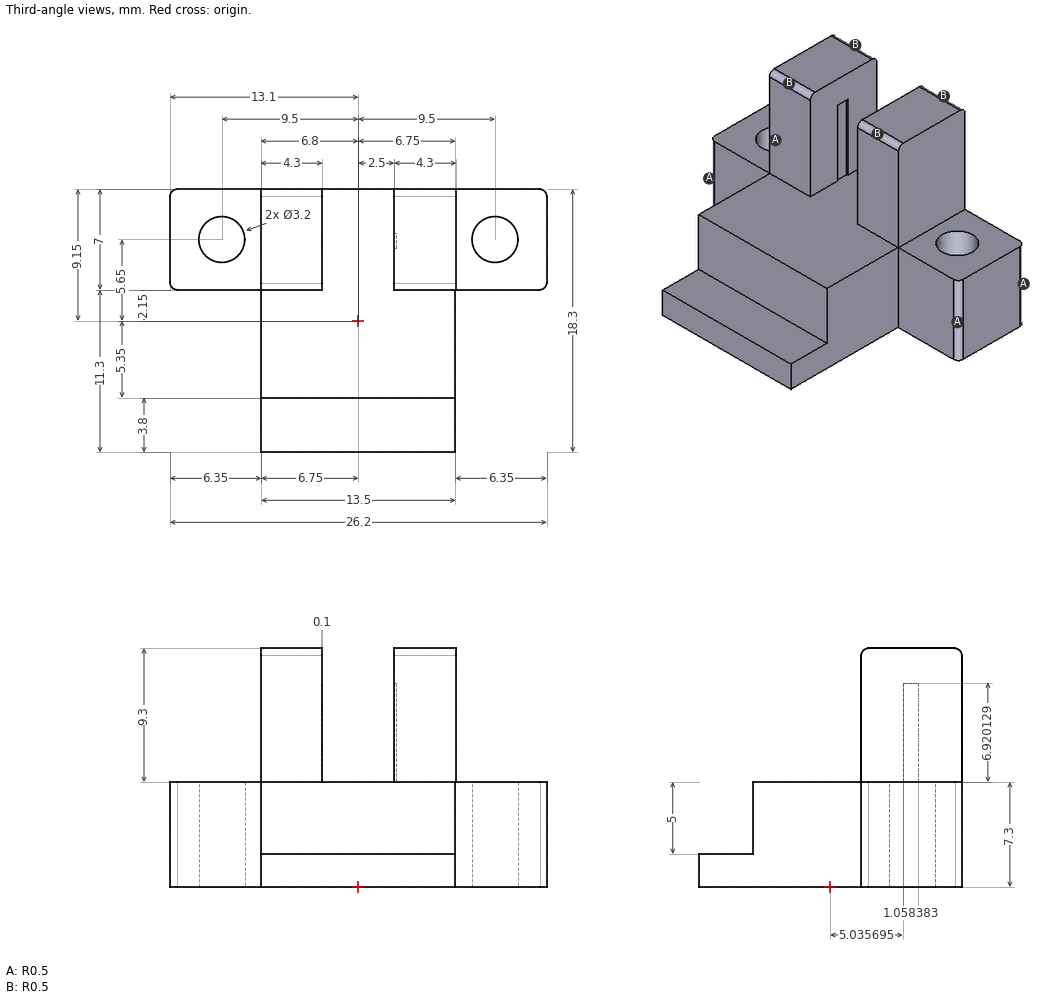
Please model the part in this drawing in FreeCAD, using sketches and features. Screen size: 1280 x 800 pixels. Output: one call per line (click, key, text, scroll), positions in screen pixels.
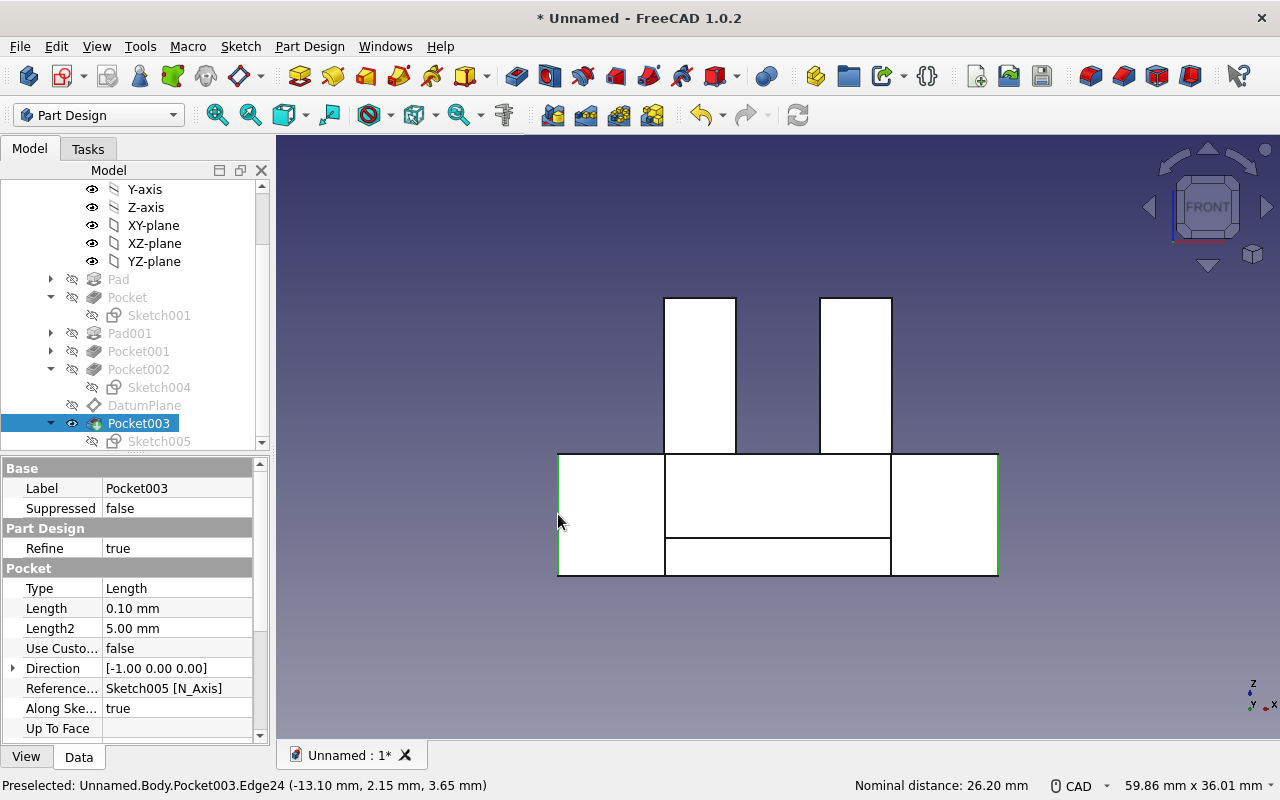
key(3)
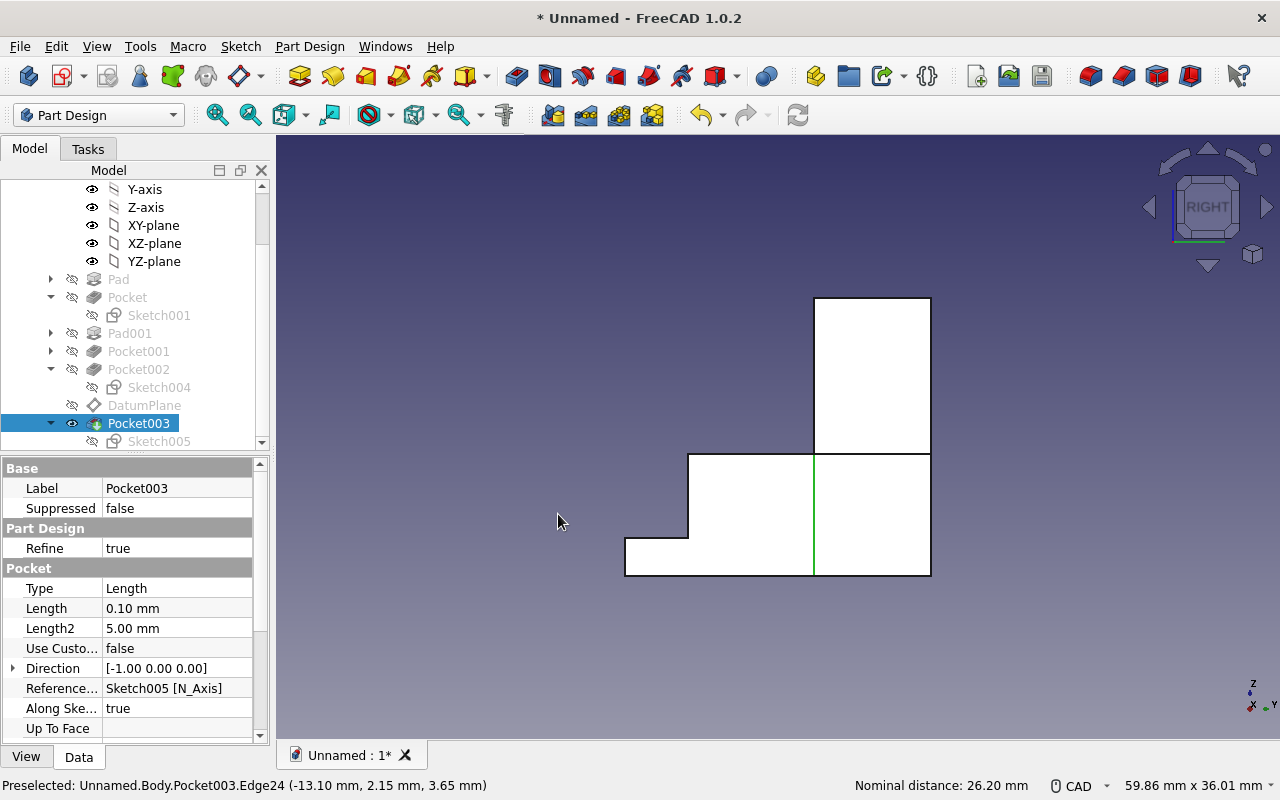
click(931, 514, ctrl)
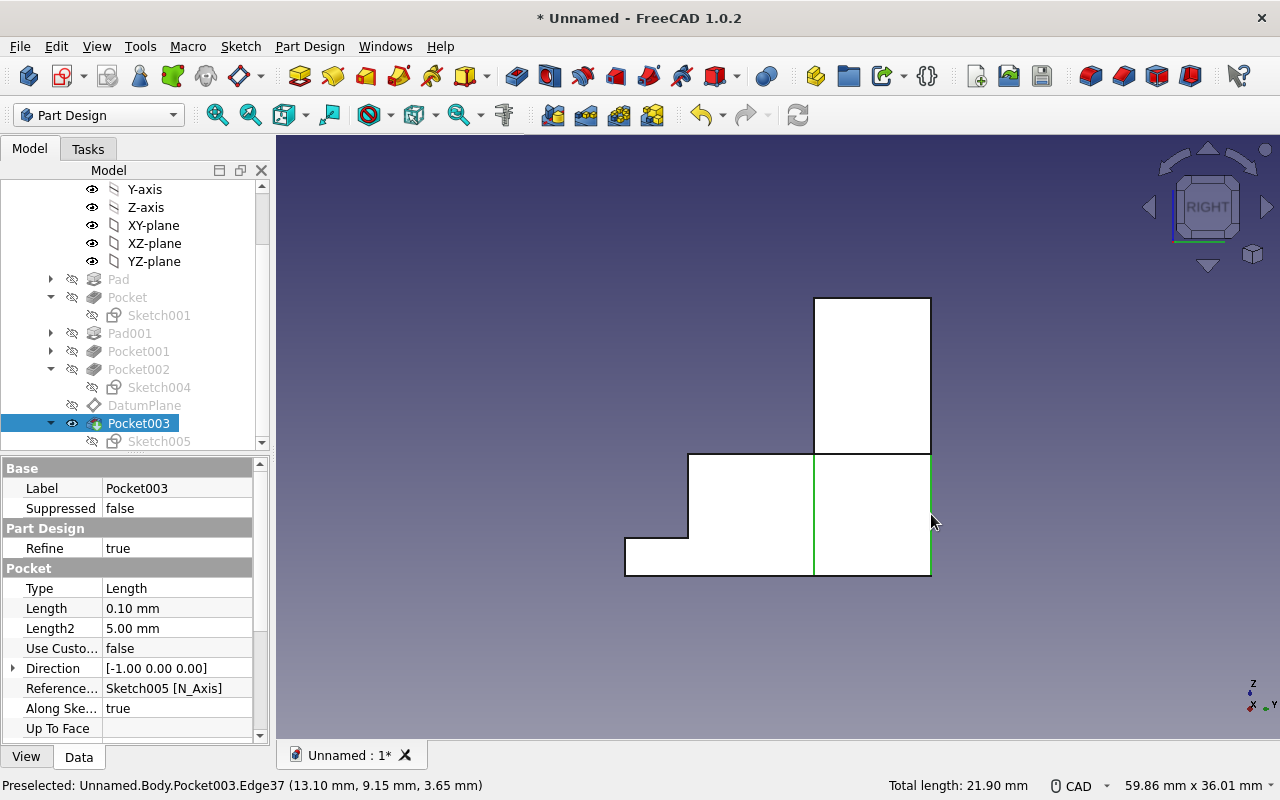
key(5)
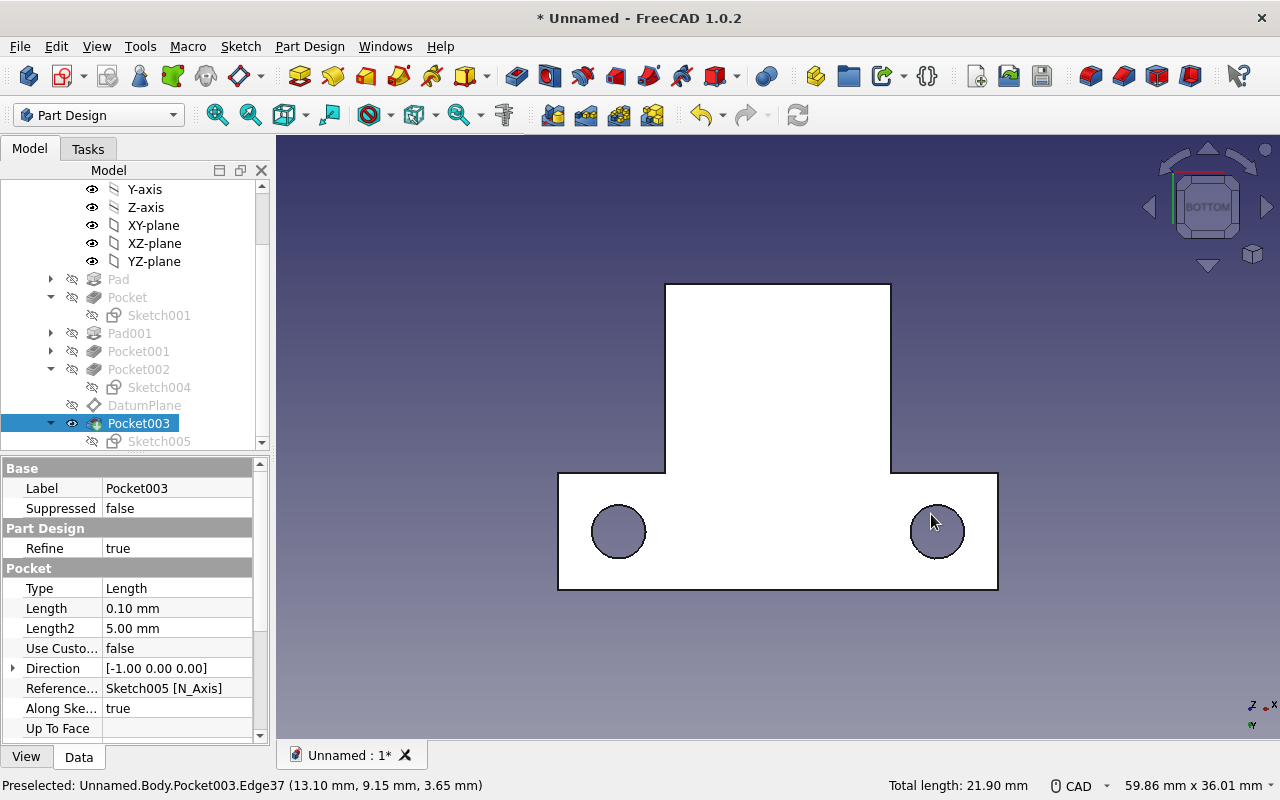
key(4)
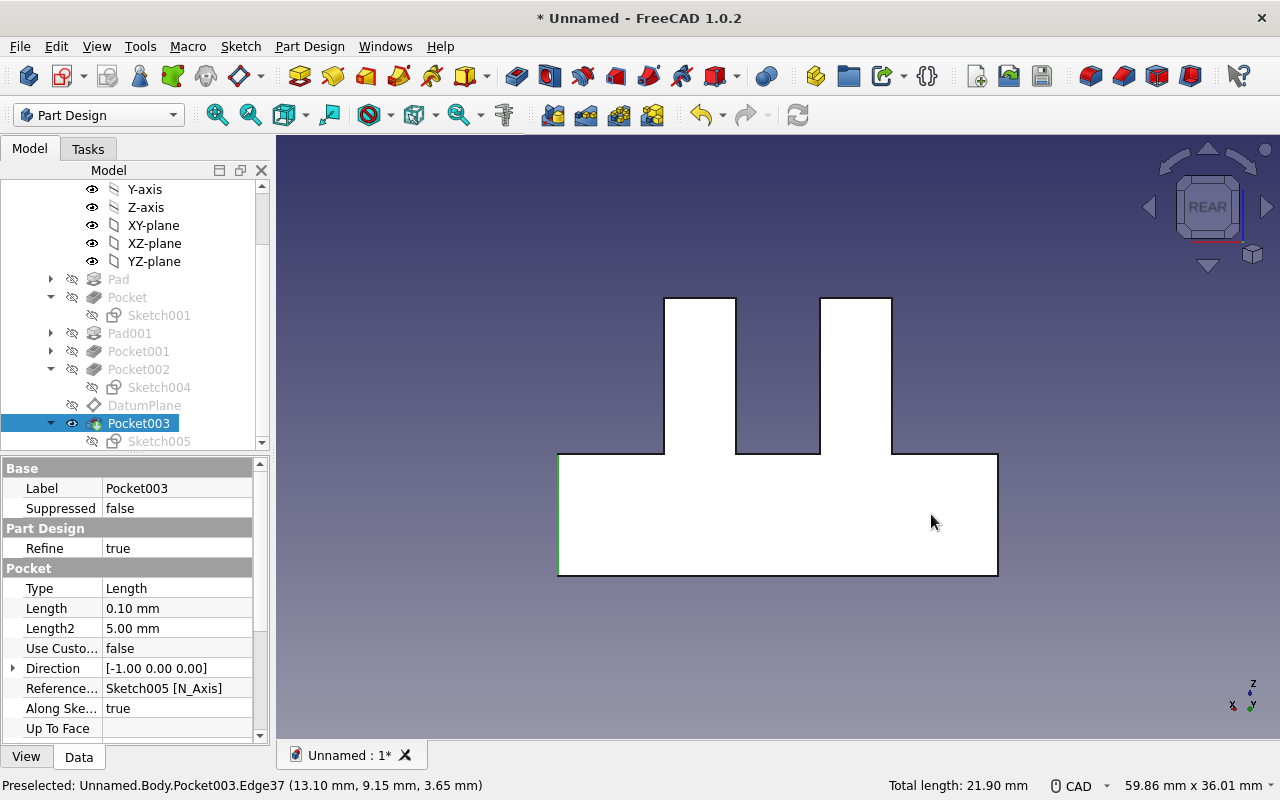
click(998, 514, ctrl)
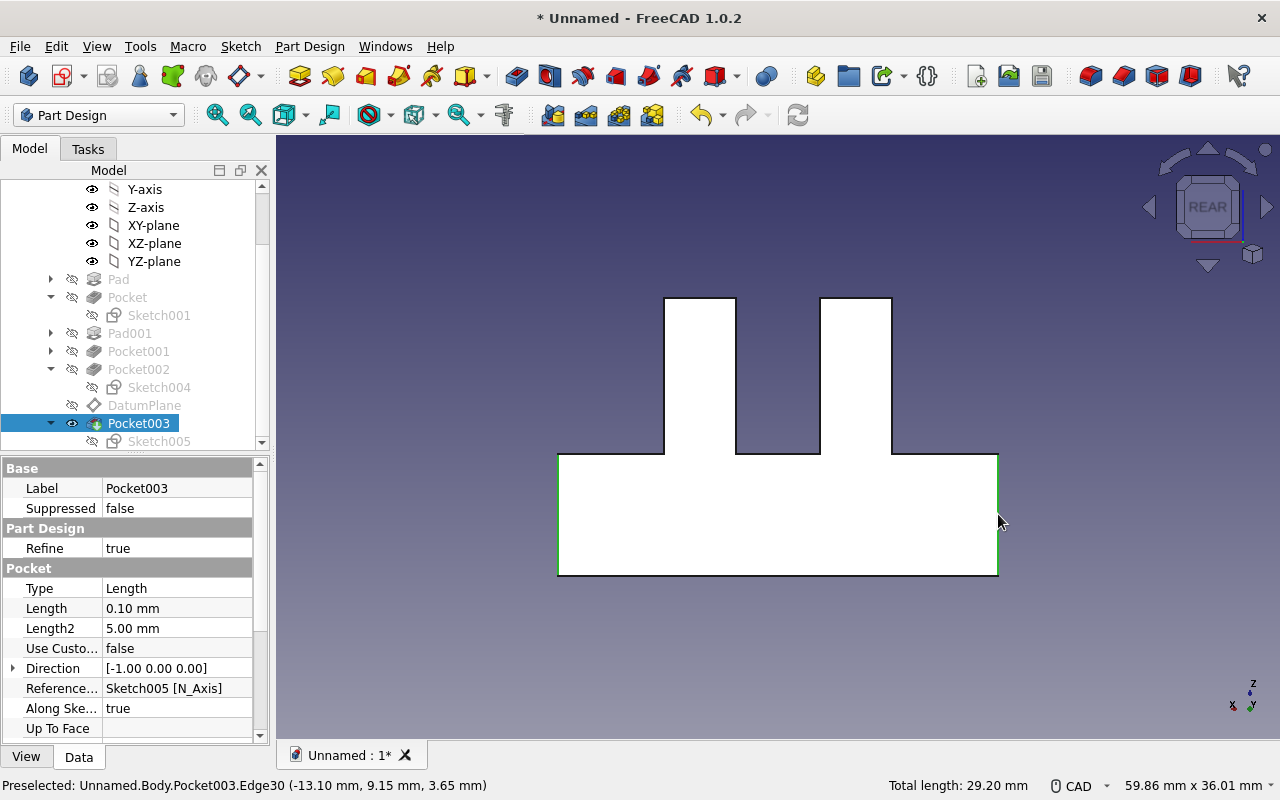
click(1091, 76)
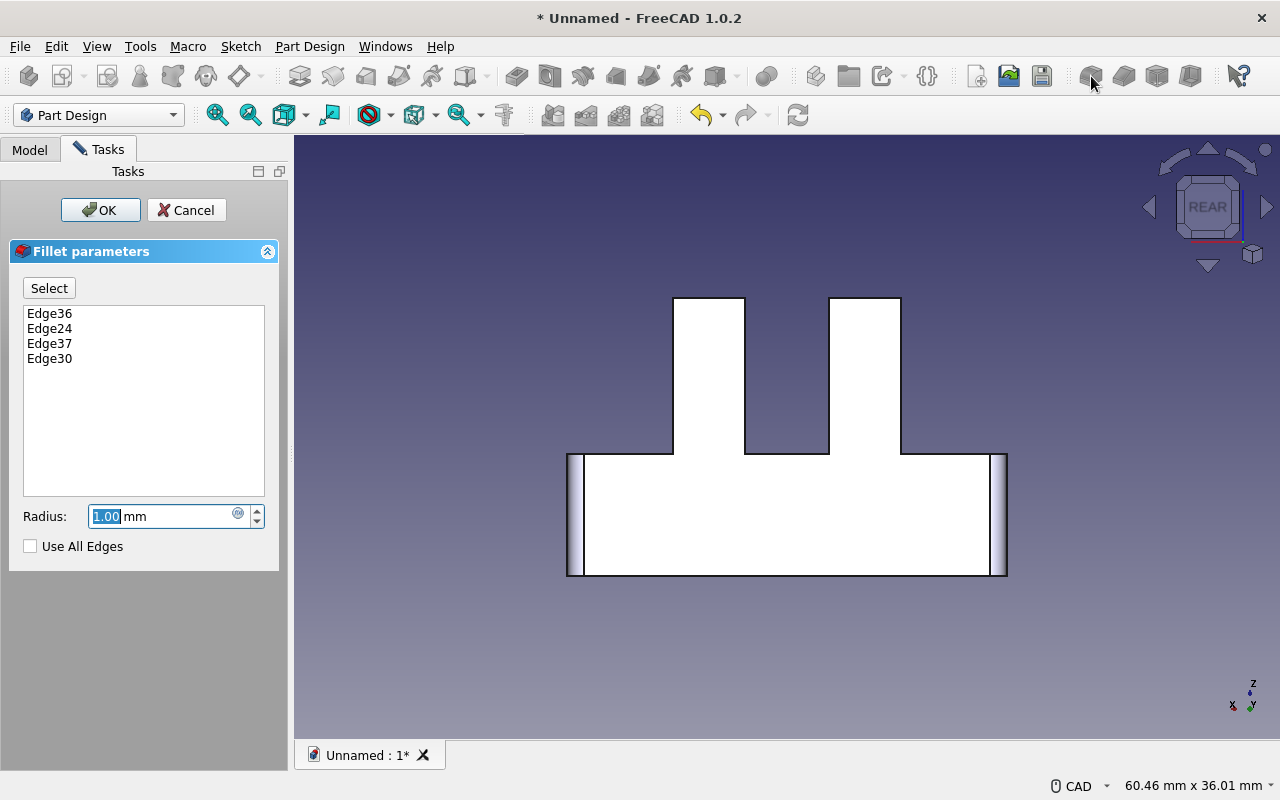
text(0.5)
key(Tab)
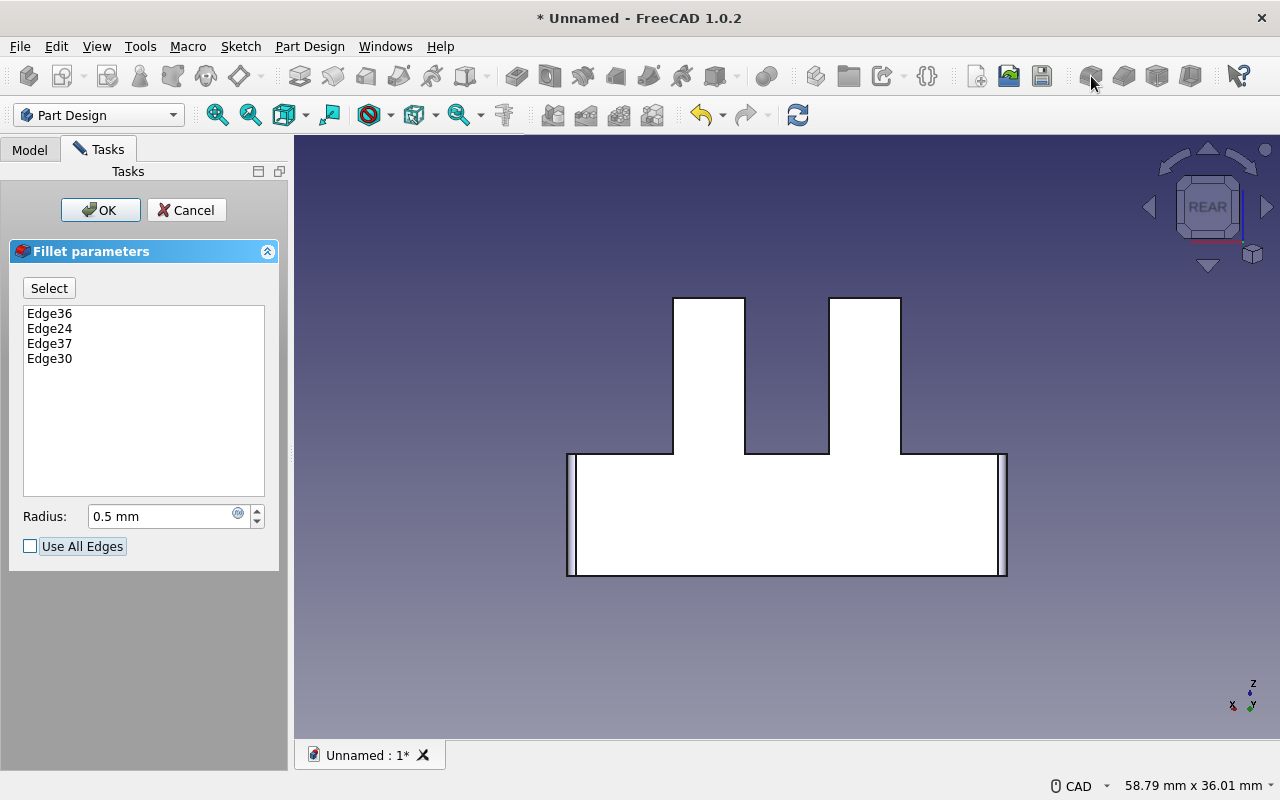
click(101, 210)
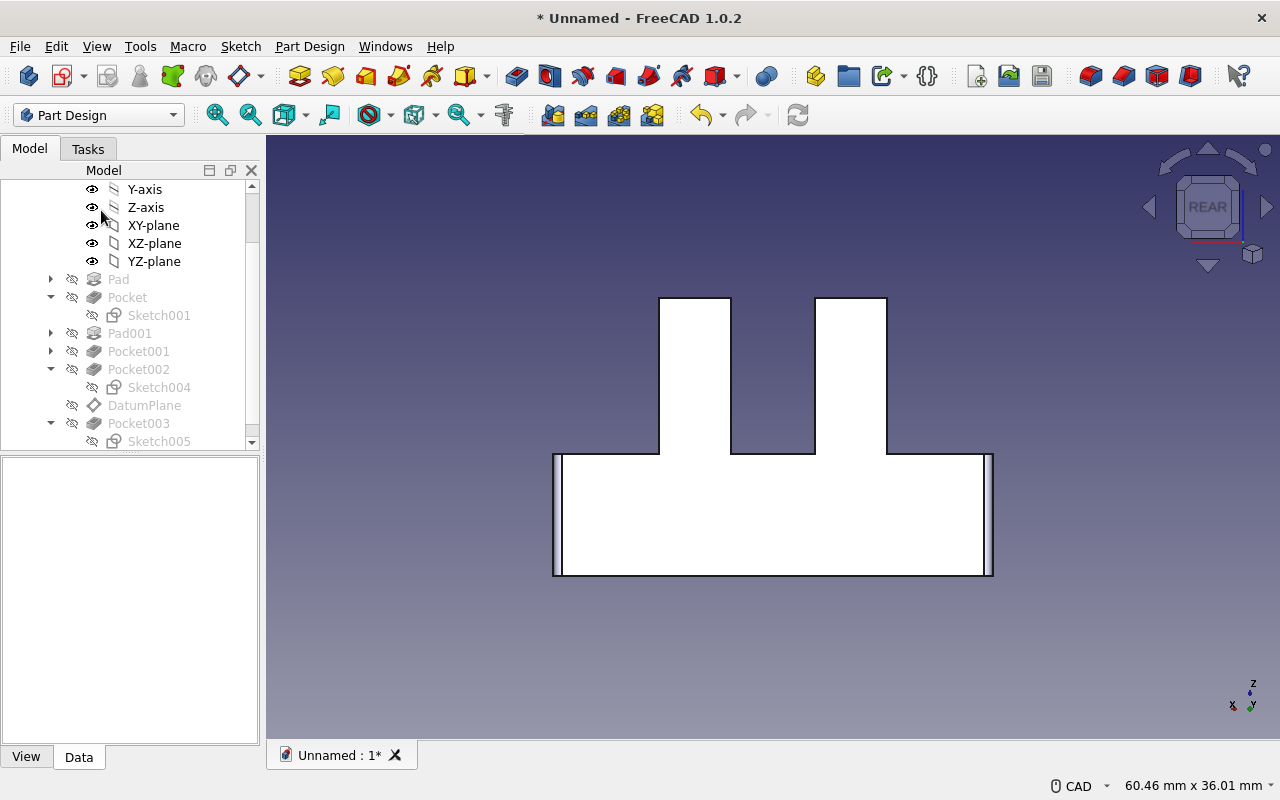
click(117, 423)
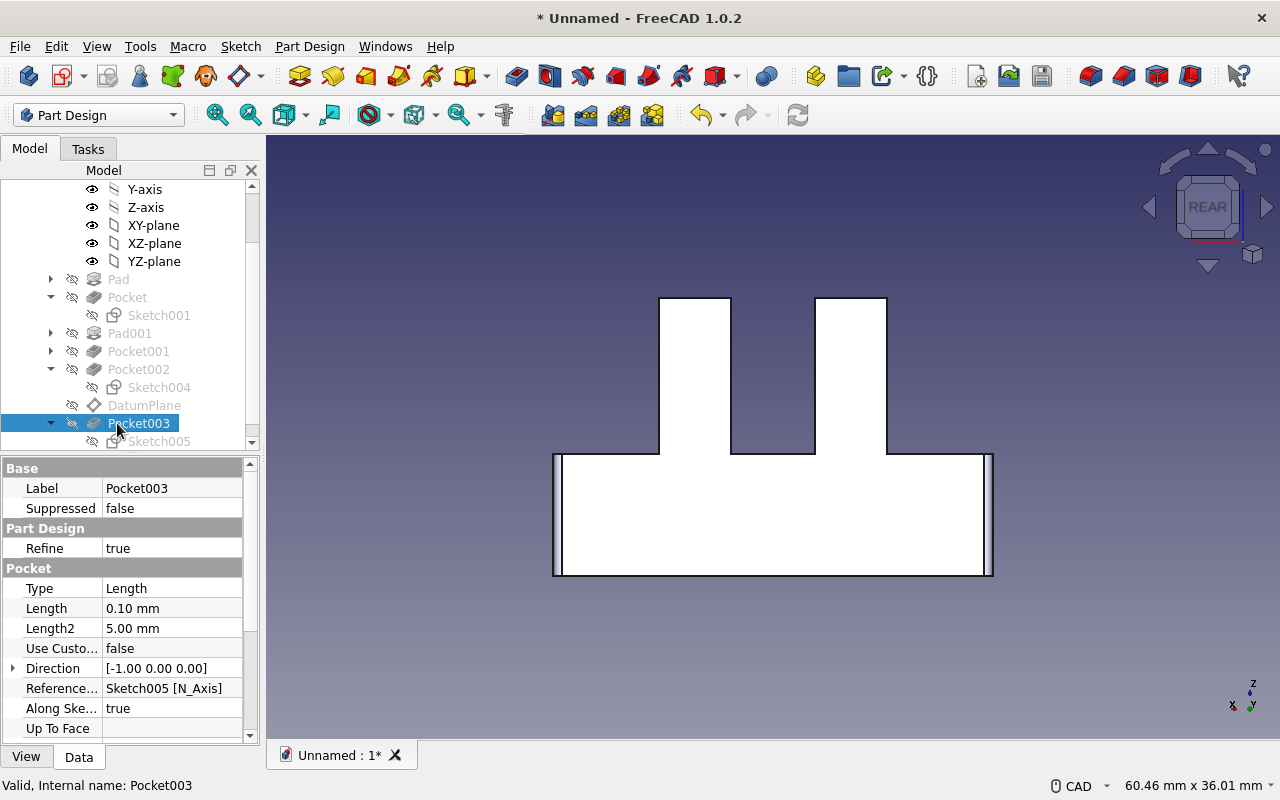
click(553, 116)